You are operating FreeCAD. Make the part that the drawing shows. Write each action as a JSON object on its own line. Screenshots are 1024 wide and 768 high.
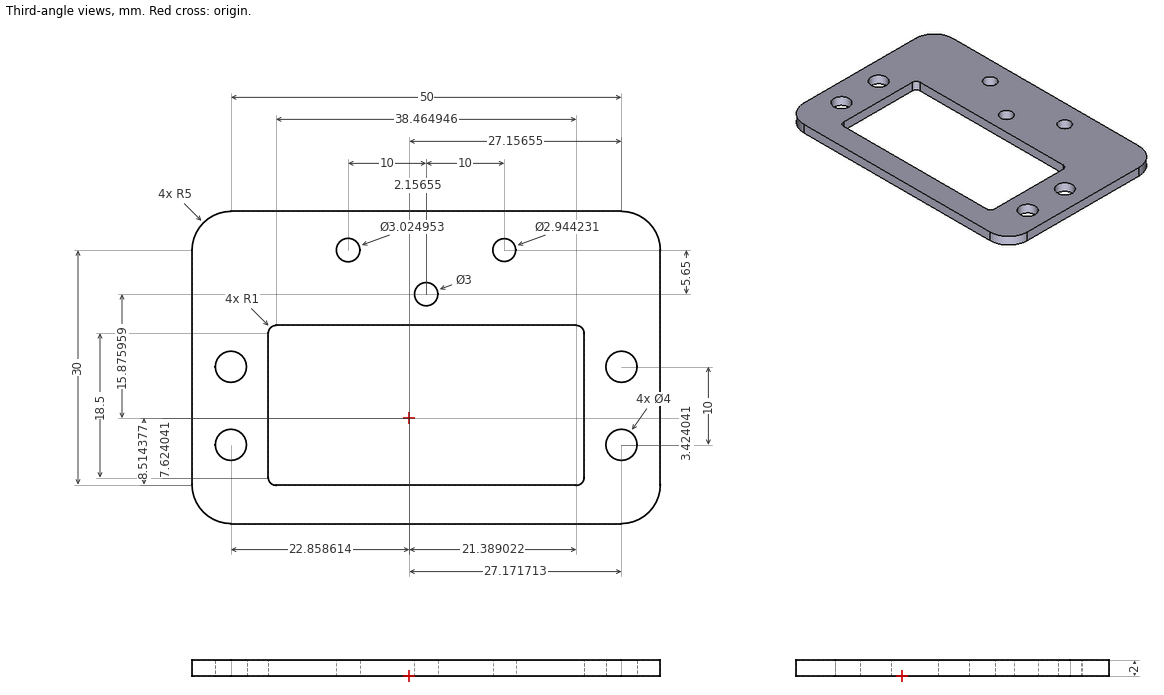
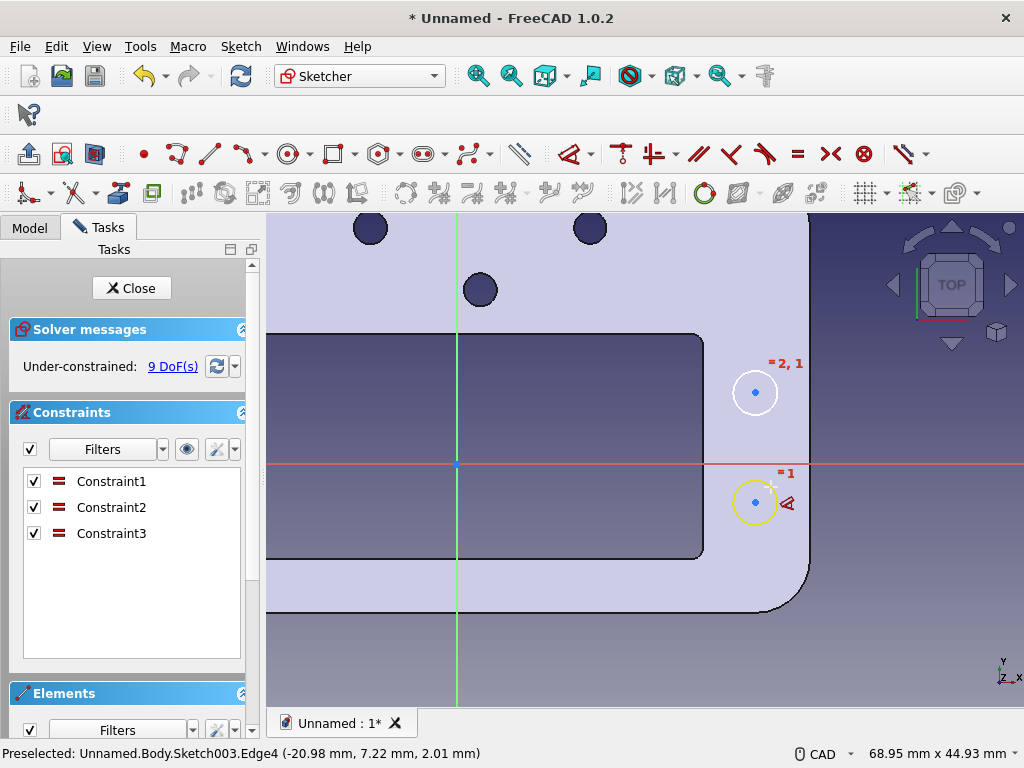
{"action": "left_click", "coordinate": [771, 487]}
{"action": "left_click", "coordinate": [807, 487]}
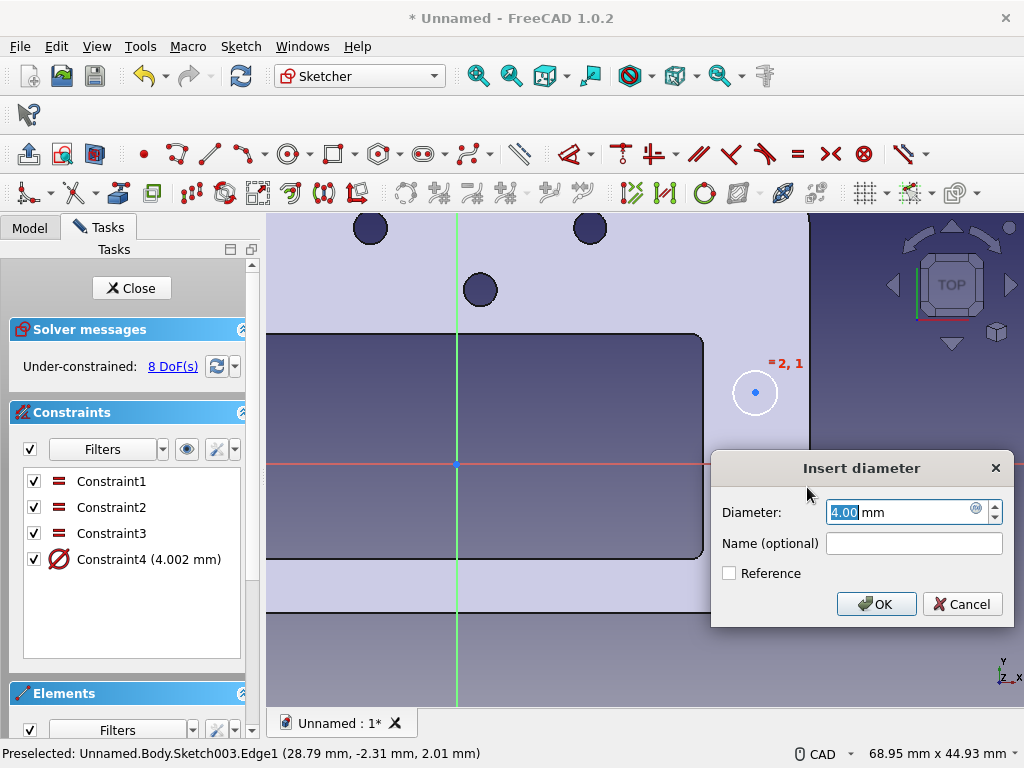
{"action": "type", "text": "4"}
{"action": "key", "text": "Return"}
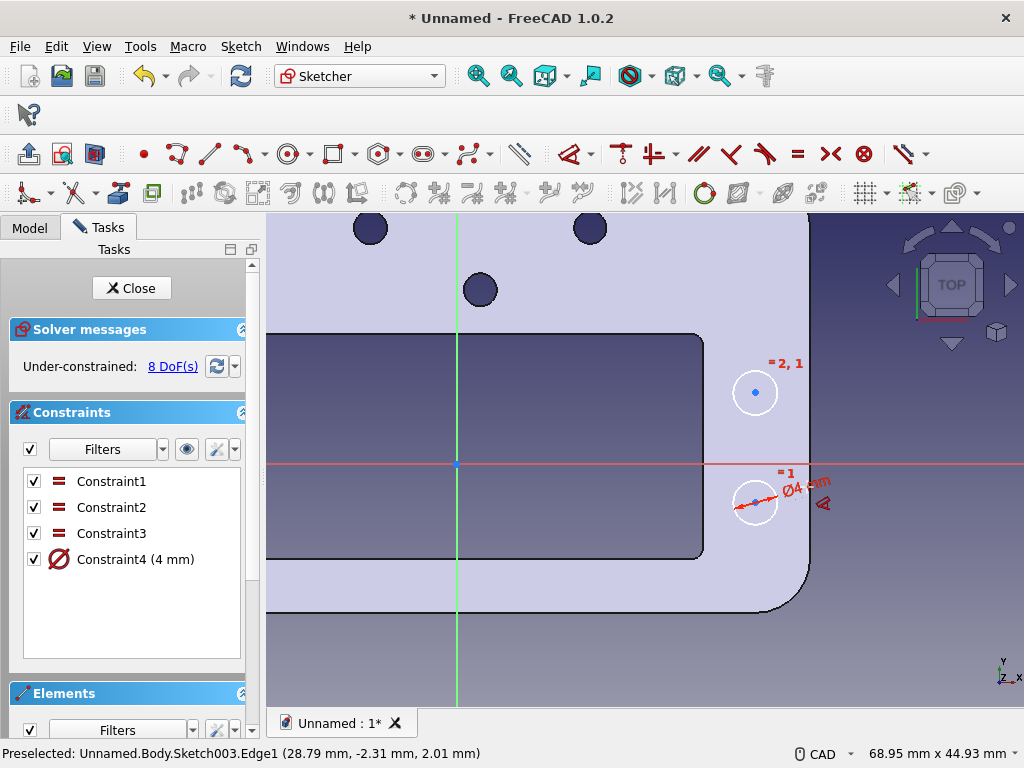
{"action": "left_click", "coordinate": [755, 503]}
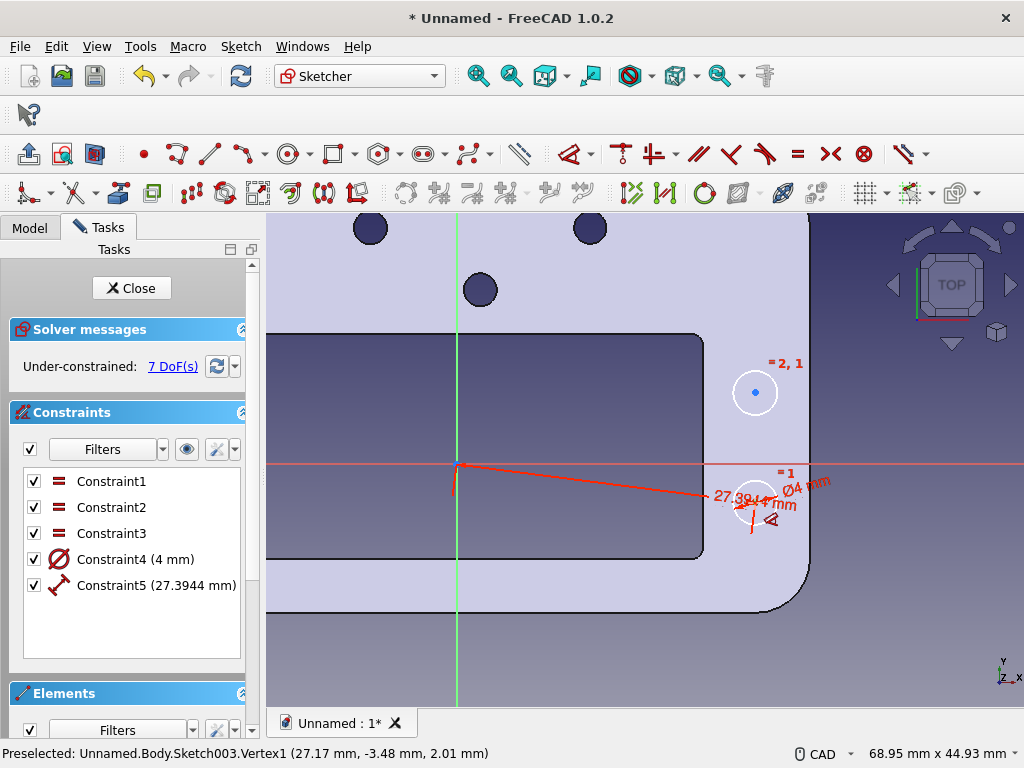
{"action": "left_click", "coordinate": [755, 393]}
{"action": "left_click", "coordinate": [789, 448]}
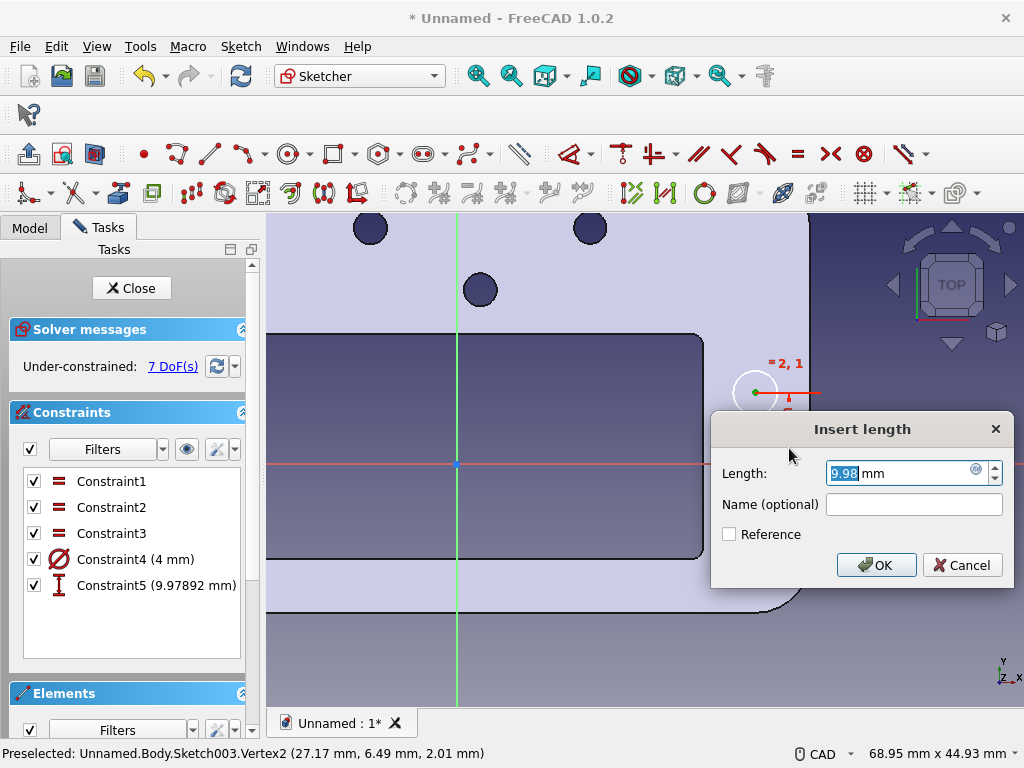
{"action": "type", "text": "10"}
{"action": "key", "text": "Return"}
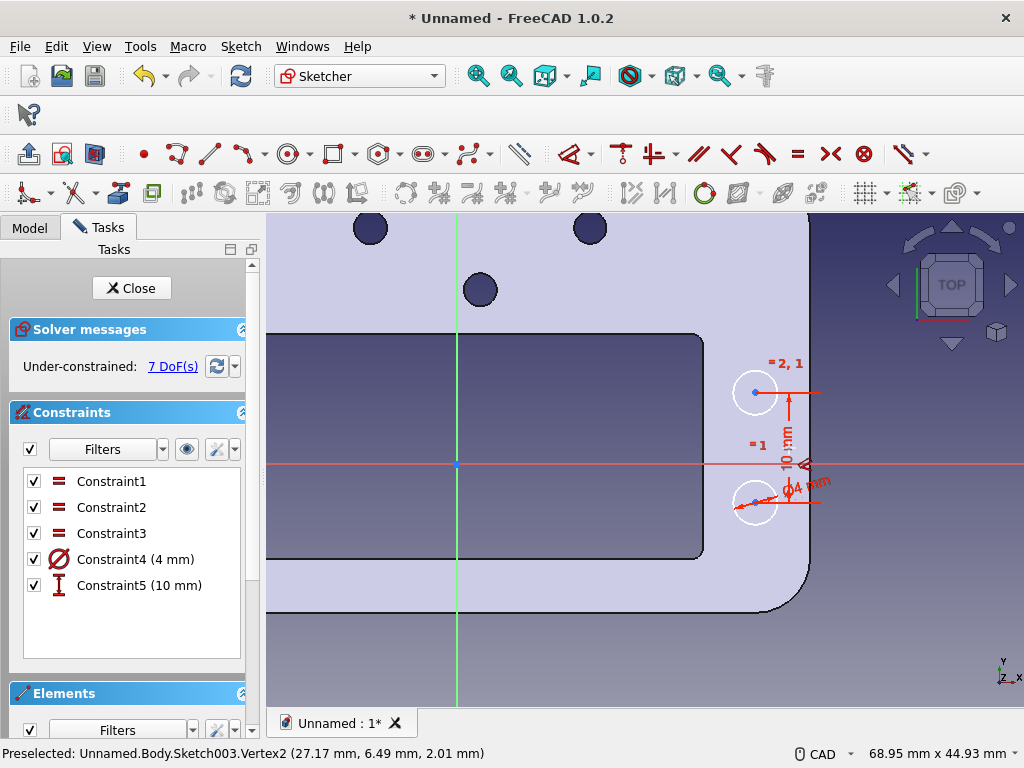
{"action": "left_click", "coordinate": [755, 393]}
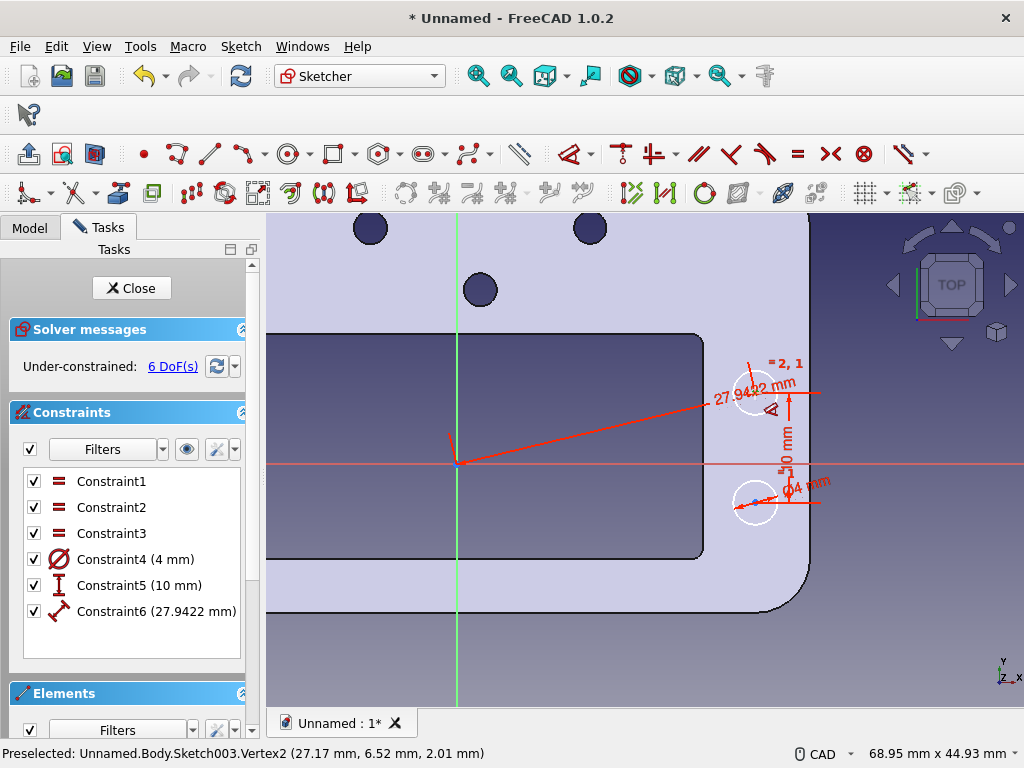
{"action": "scroll", "coordinate": [772, 486], "scroll_direction": "down", "scroll_amount": 2}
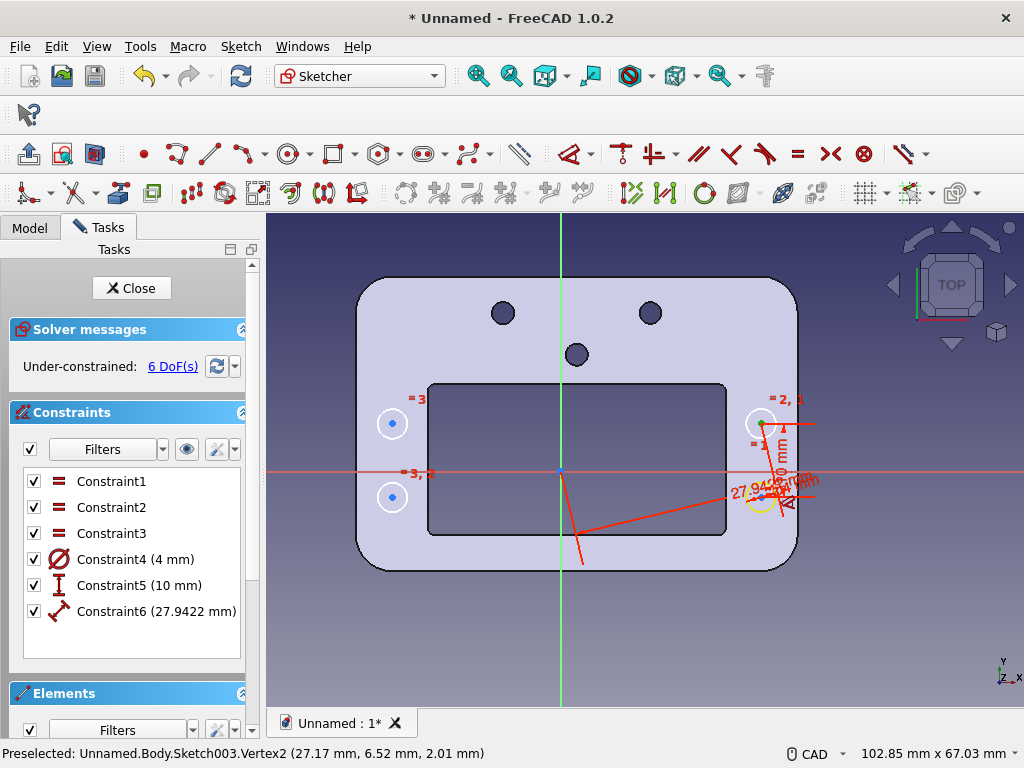
{"action": "left_click", "coordinate": [393, 497]}
{"action": "left_click", "coordinate": [795, 435]}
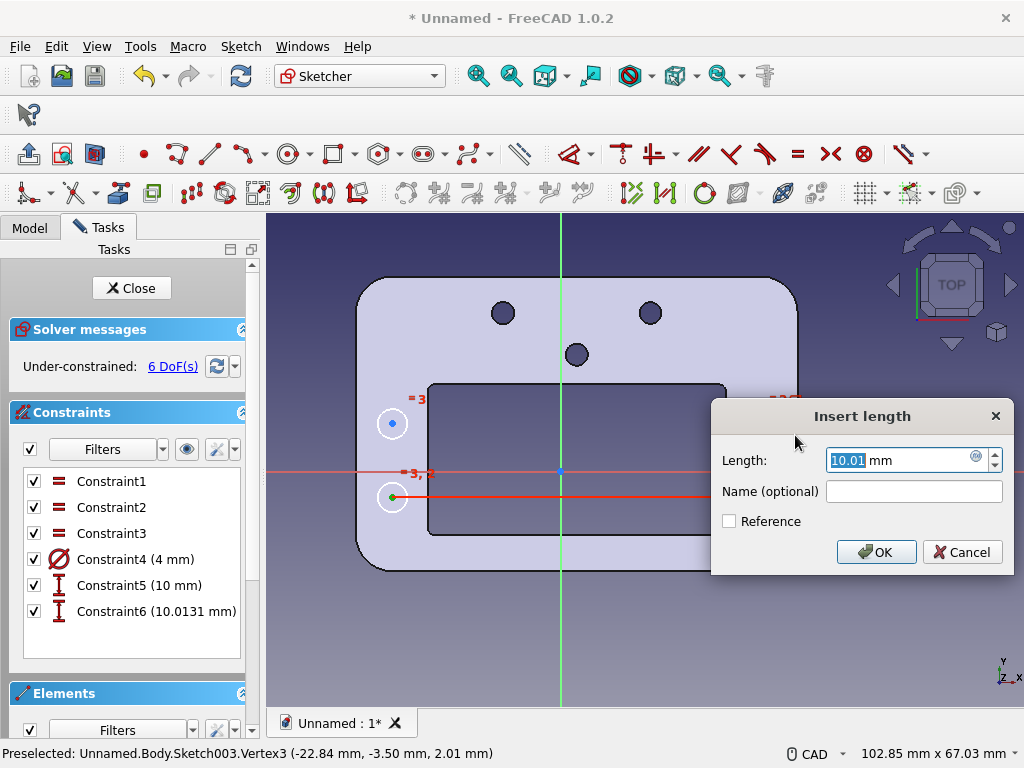
{"action": "type", "text": "10"}
{"action": "key", "text": "Return"}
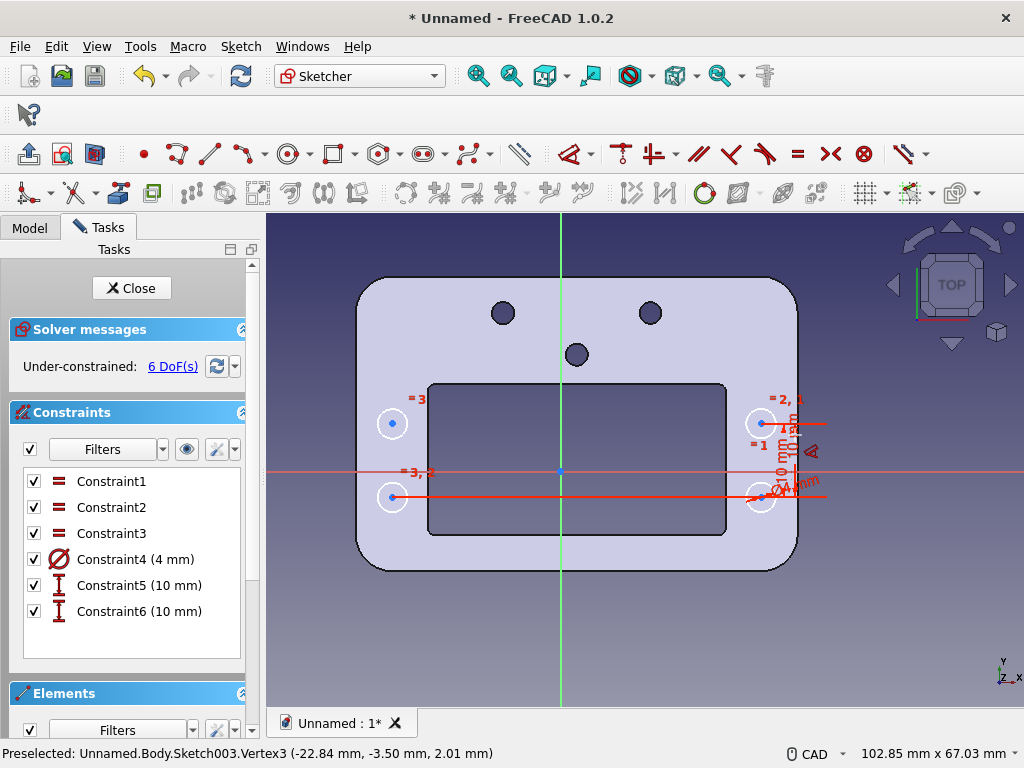
{"action": "left_click", "coordinate": [393, 497]}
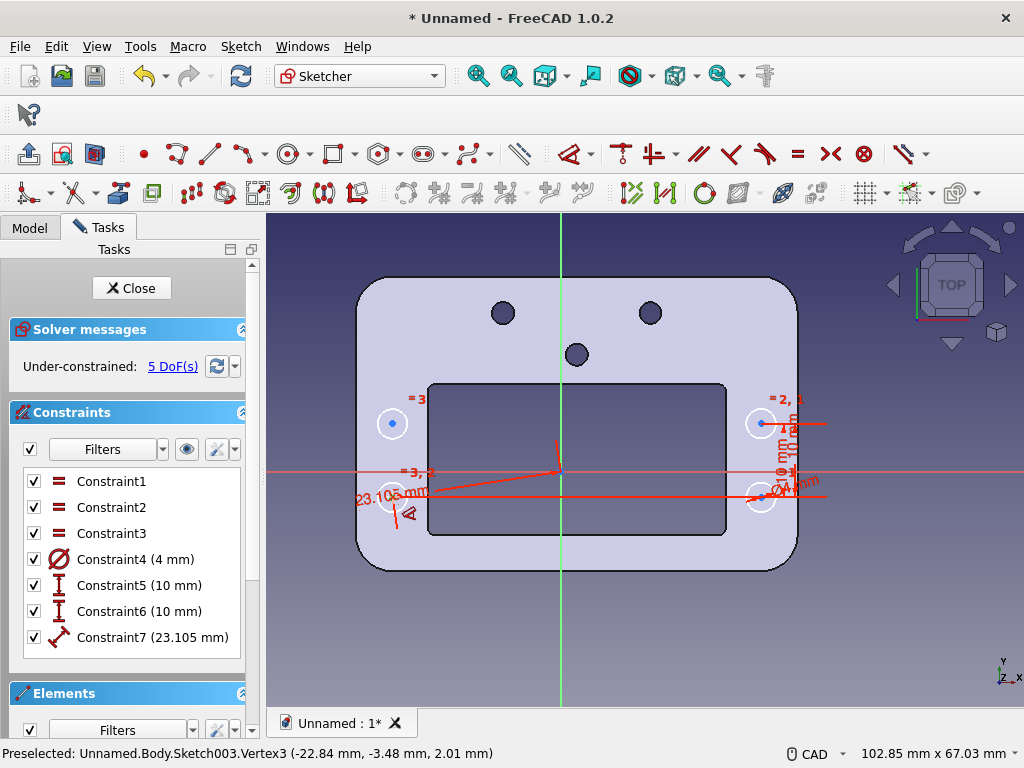
{"action": "left_click", "coordinate": [393, 424]}
{"action": "left_click", "coordinate": [359, 444]}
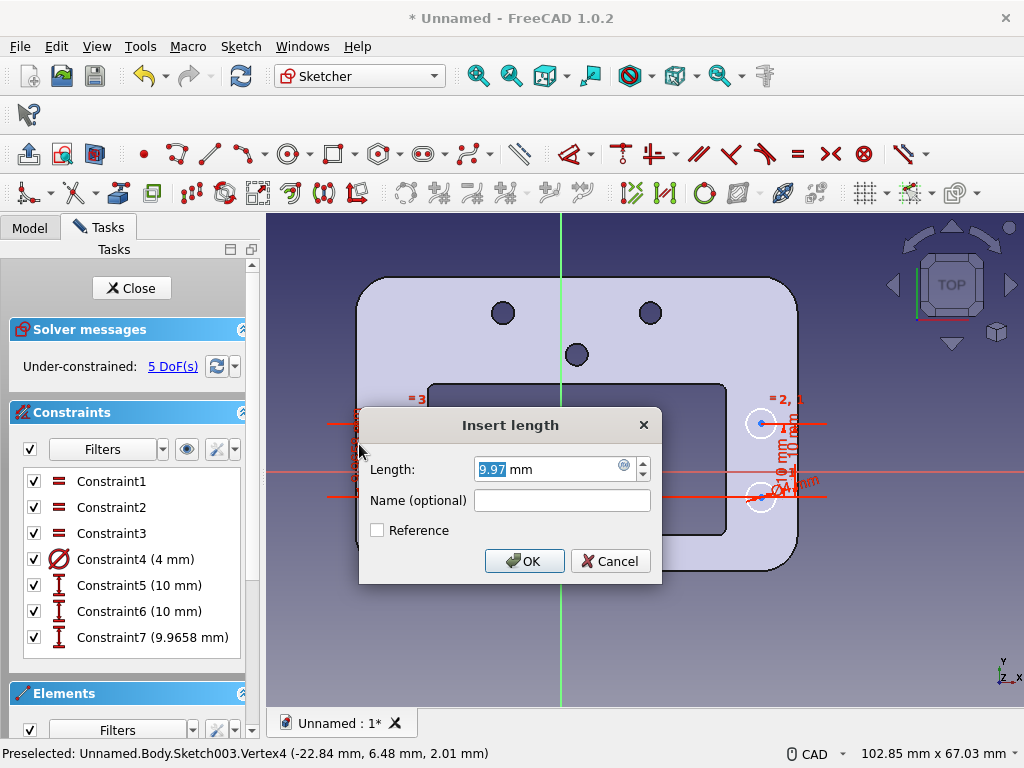
{"action": "type", "text": "10"}
{"action": "key", "text": "Return"}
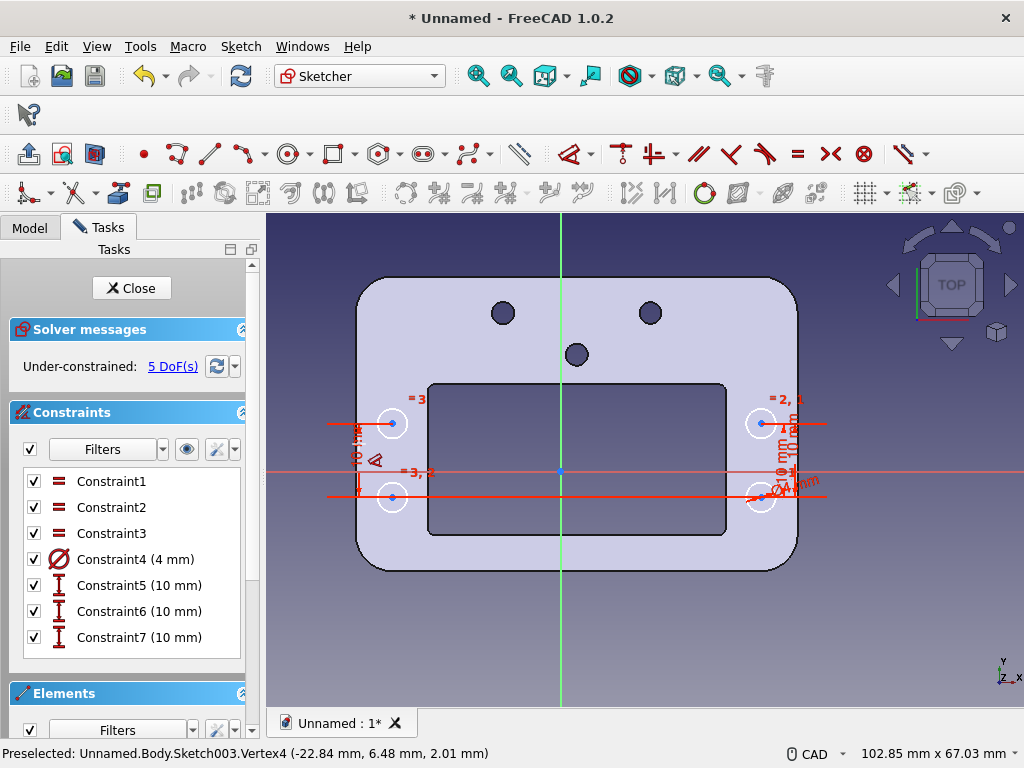
{"action": "scroll", "coordinate": [761, 497], "scroll_direction": "up", "scroll_amount": 3}